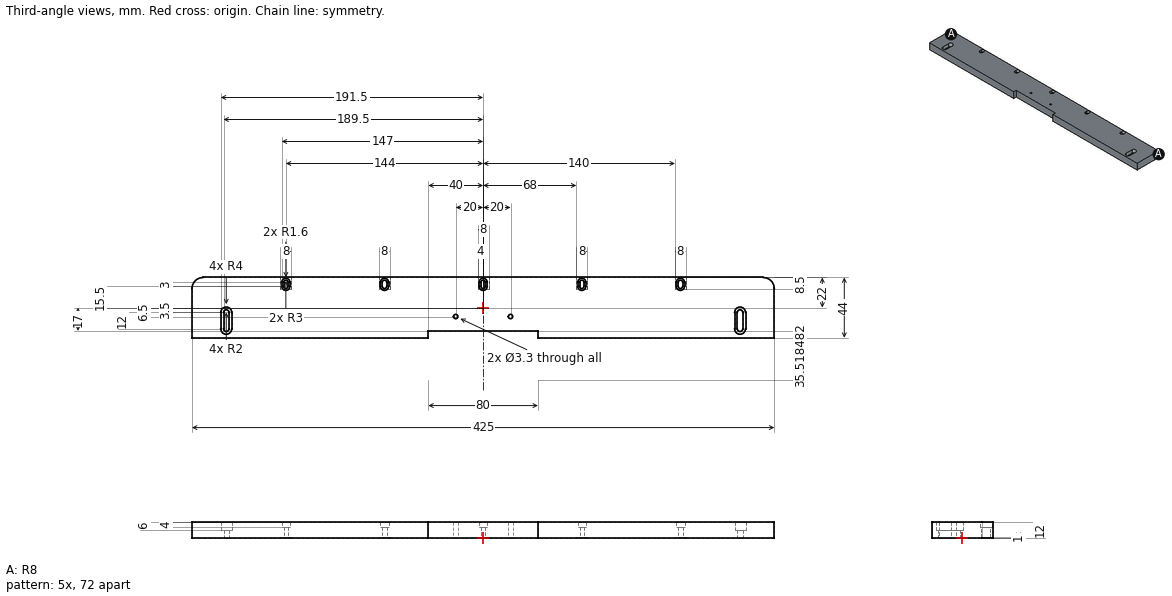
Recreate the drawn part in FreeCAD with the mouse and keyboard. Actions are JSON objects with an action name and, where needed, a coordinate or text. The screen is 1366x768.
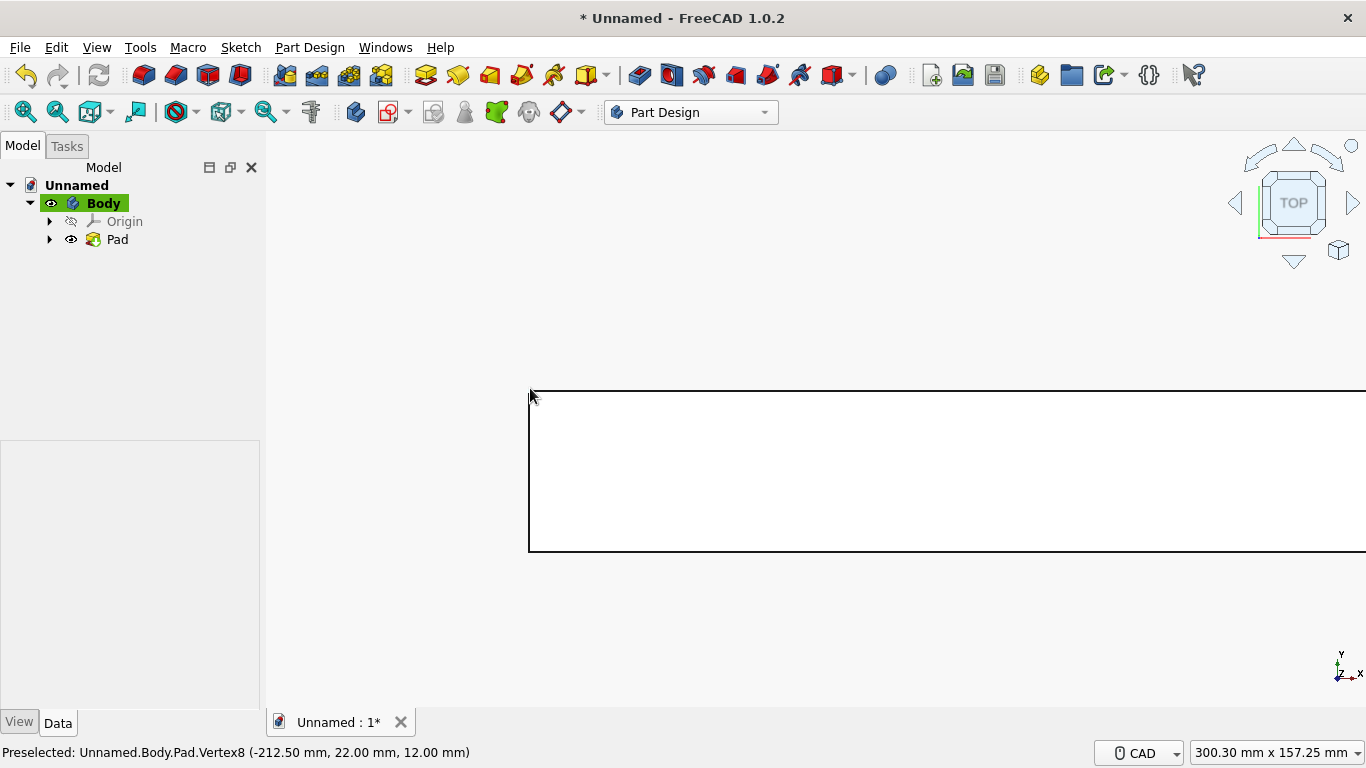
{"action": "key", "text": "v f"}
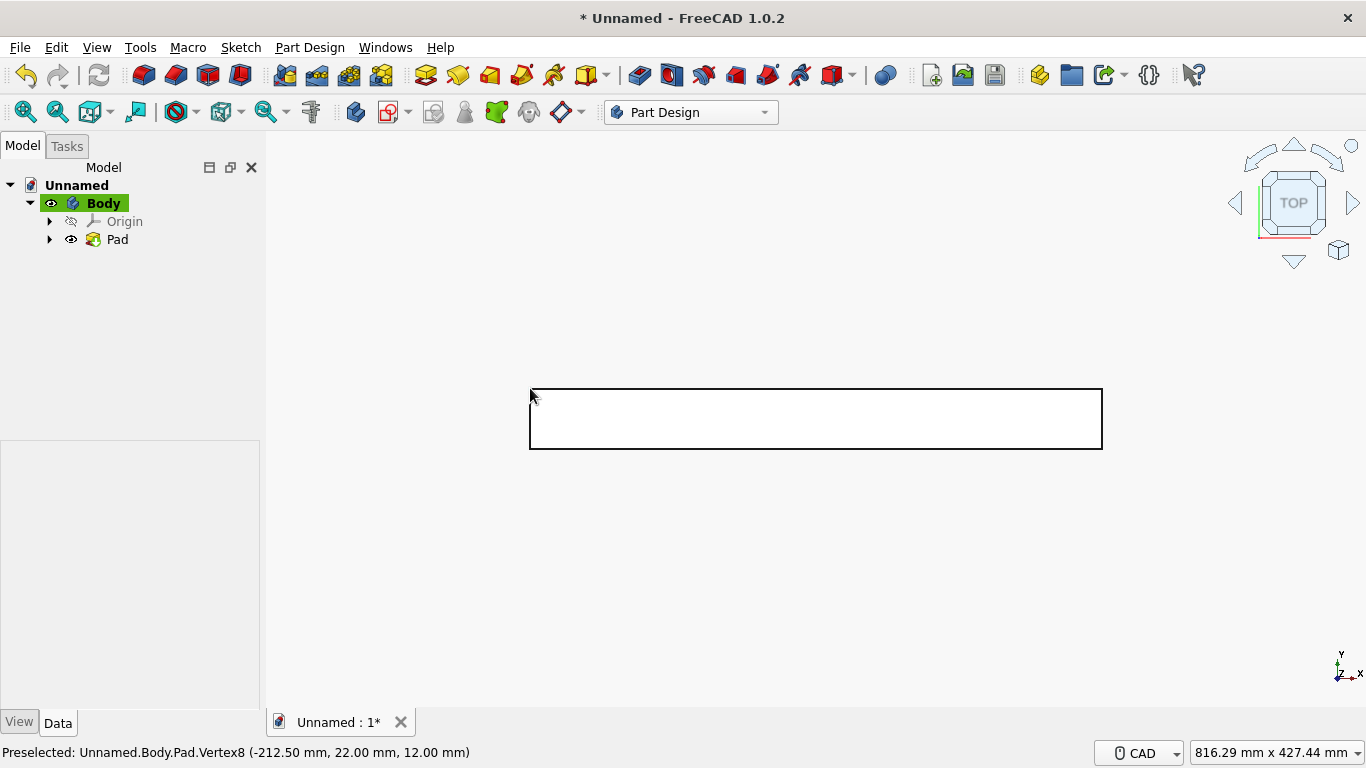
{"action": "key", "text": "1"}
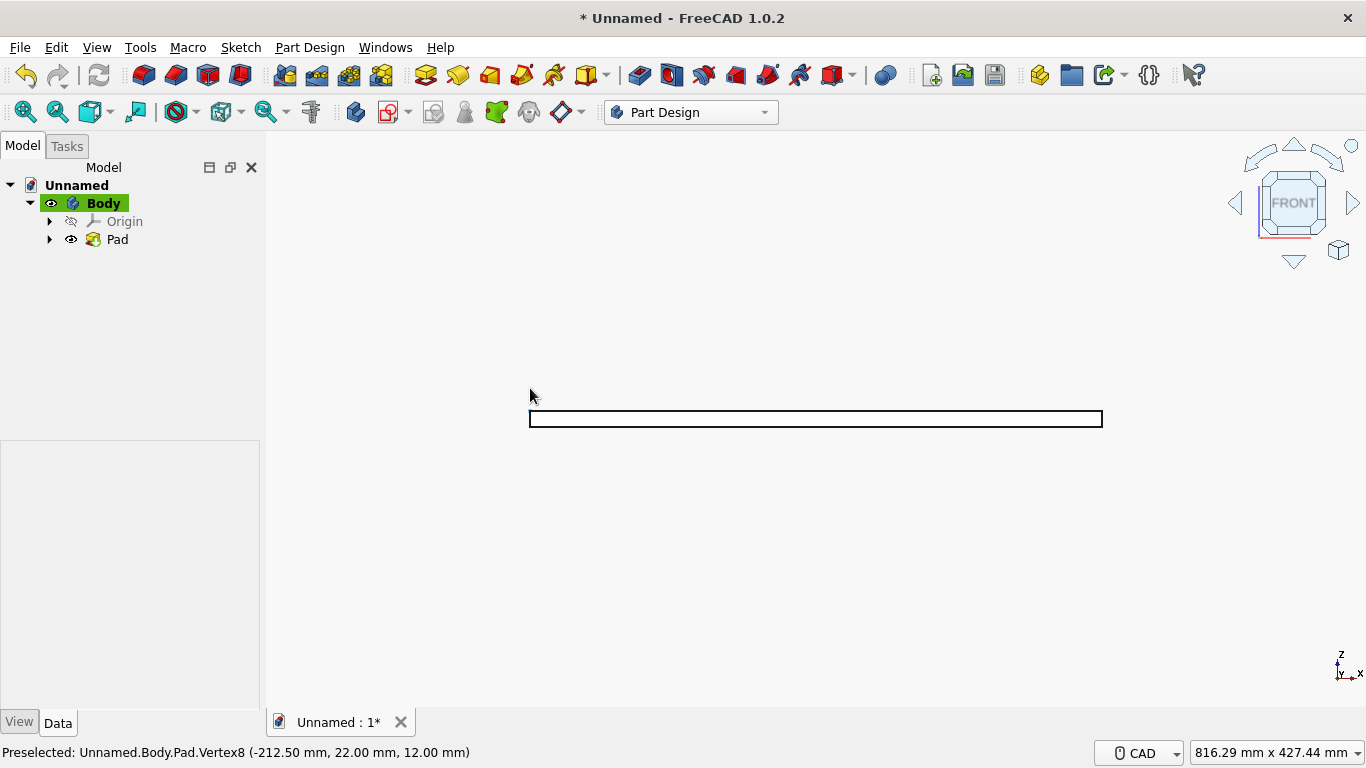
{"action": "scroll", "coordinate": [530, 418], "scroll_direction": "up", "scroll_amount": 5}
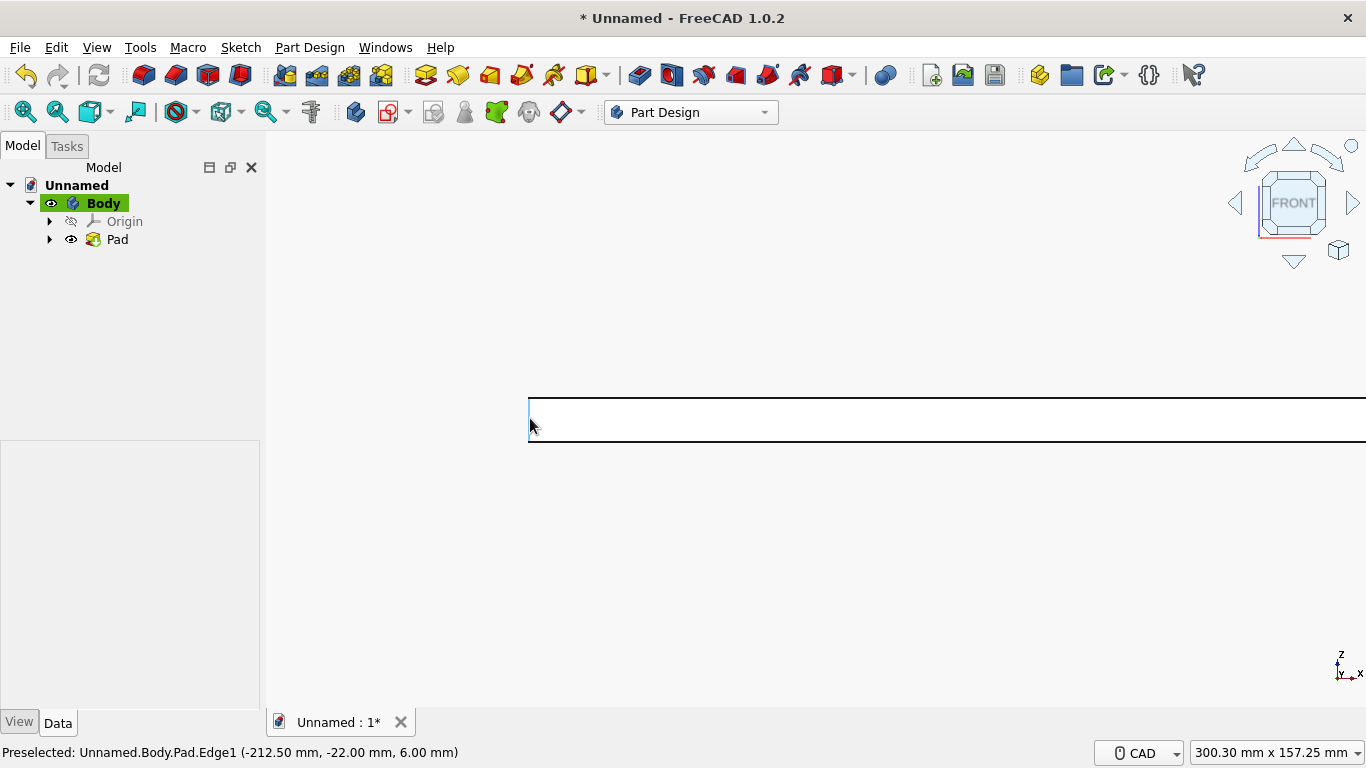
{"action": "left_click", "coordinate": [26, 112]}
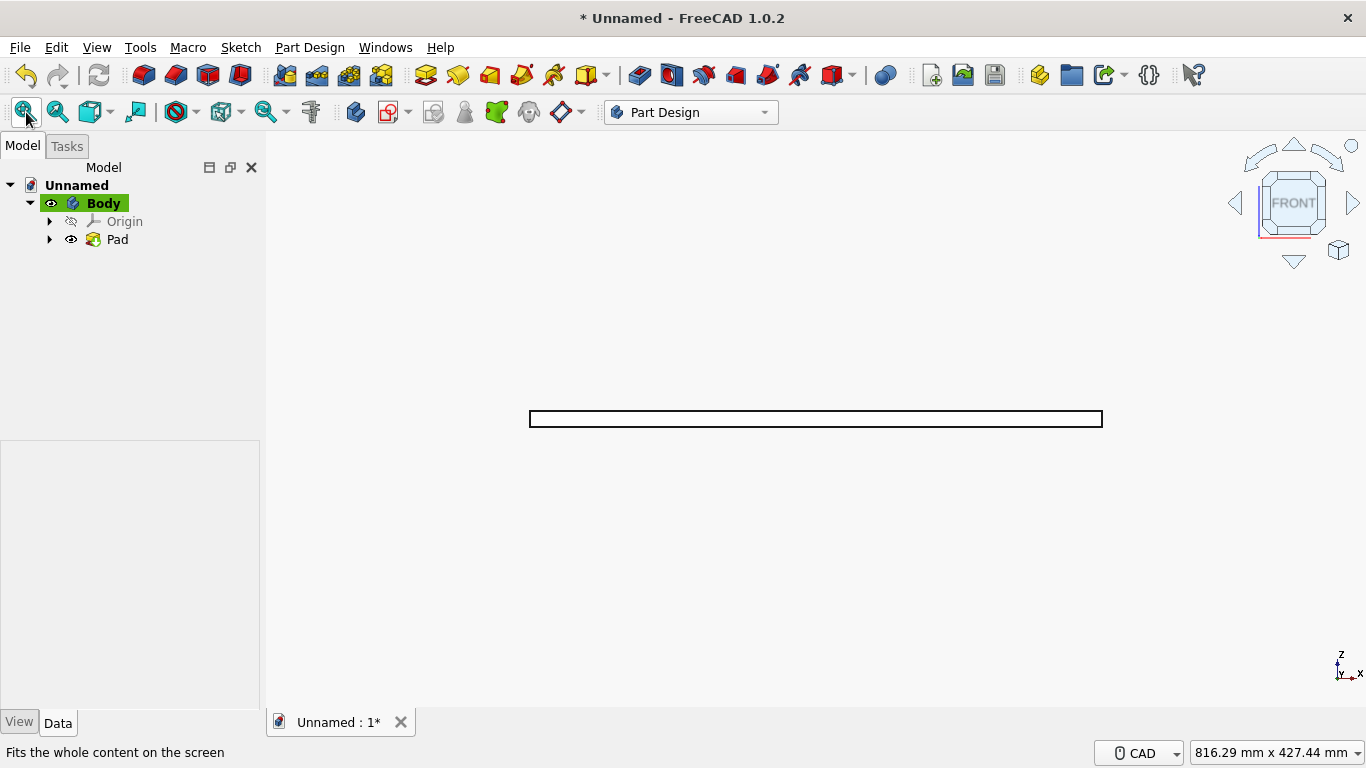
{"action": "key", "text": "3"}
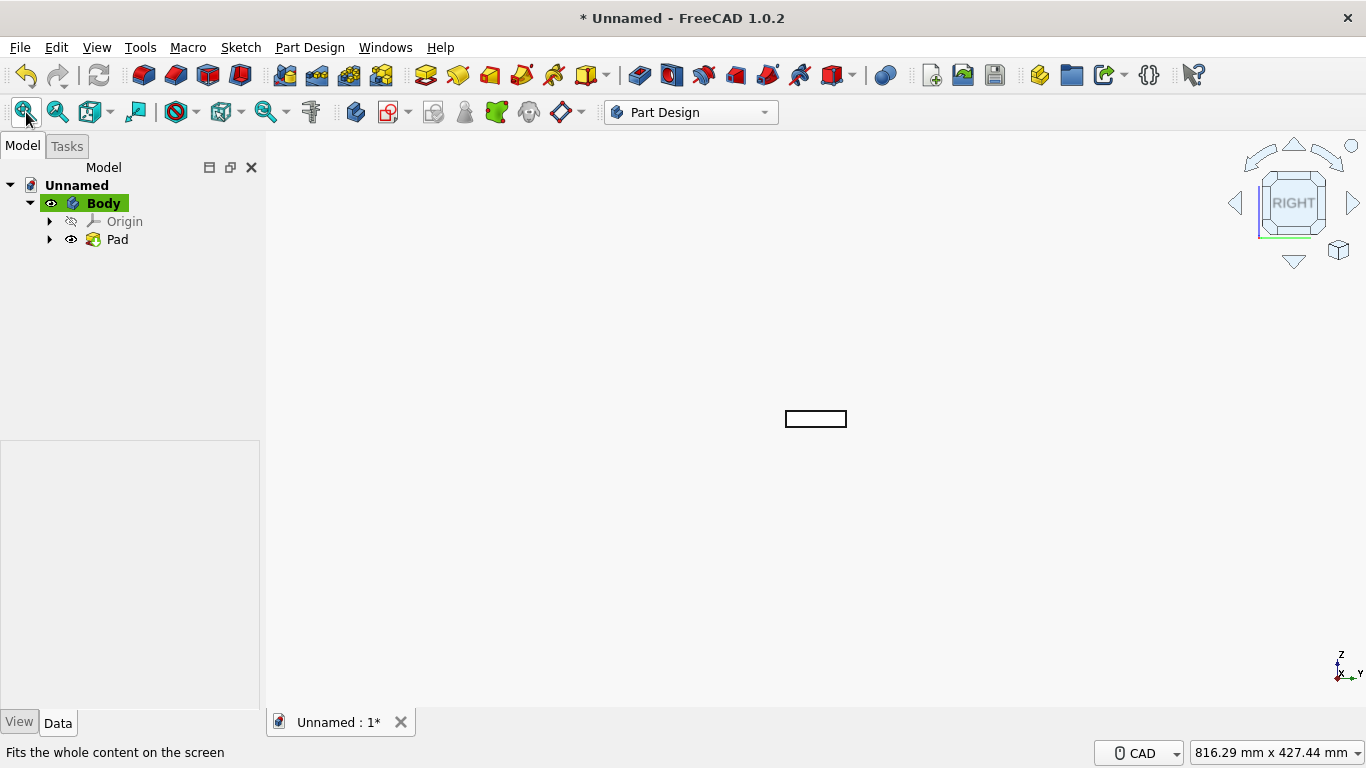
{"action": "left_click", "coordinate": [26, 112]}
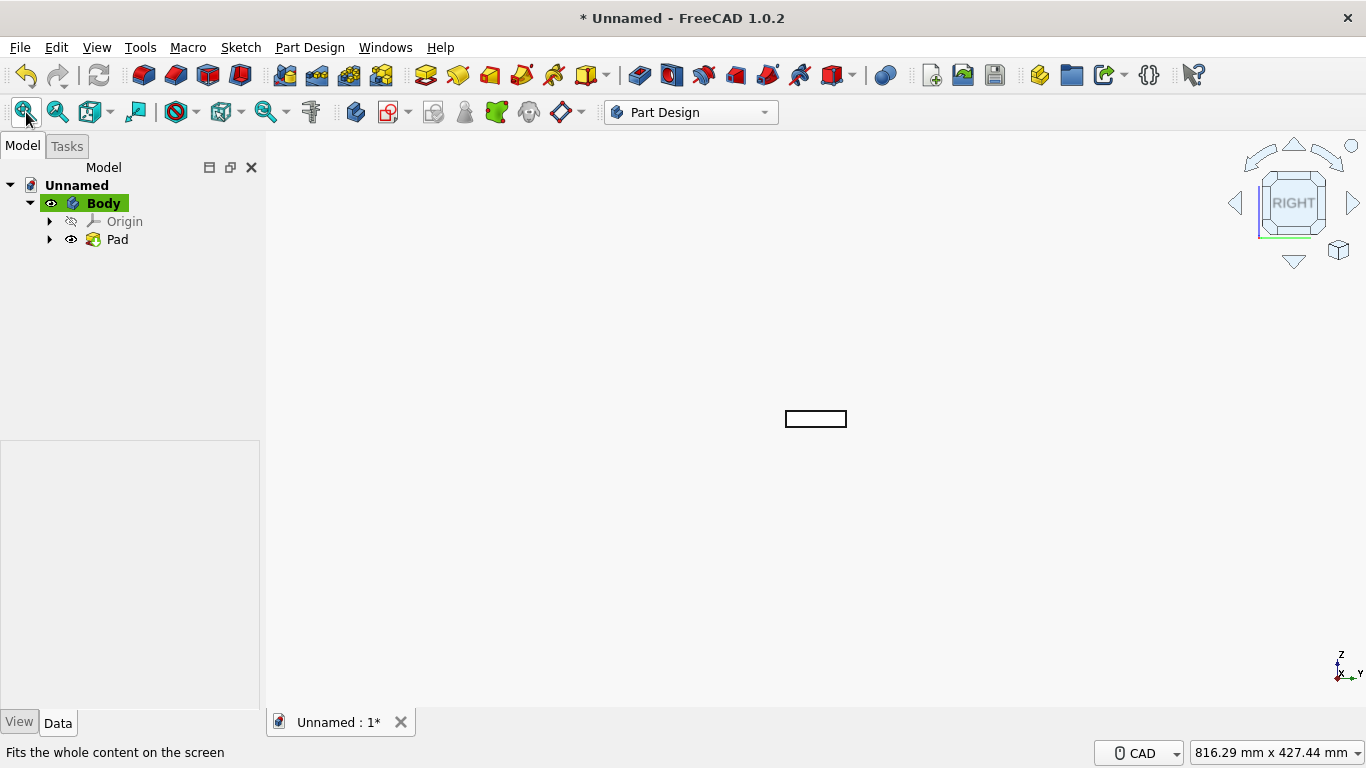
{"action": "left_click", "coordinate": [846, 418]}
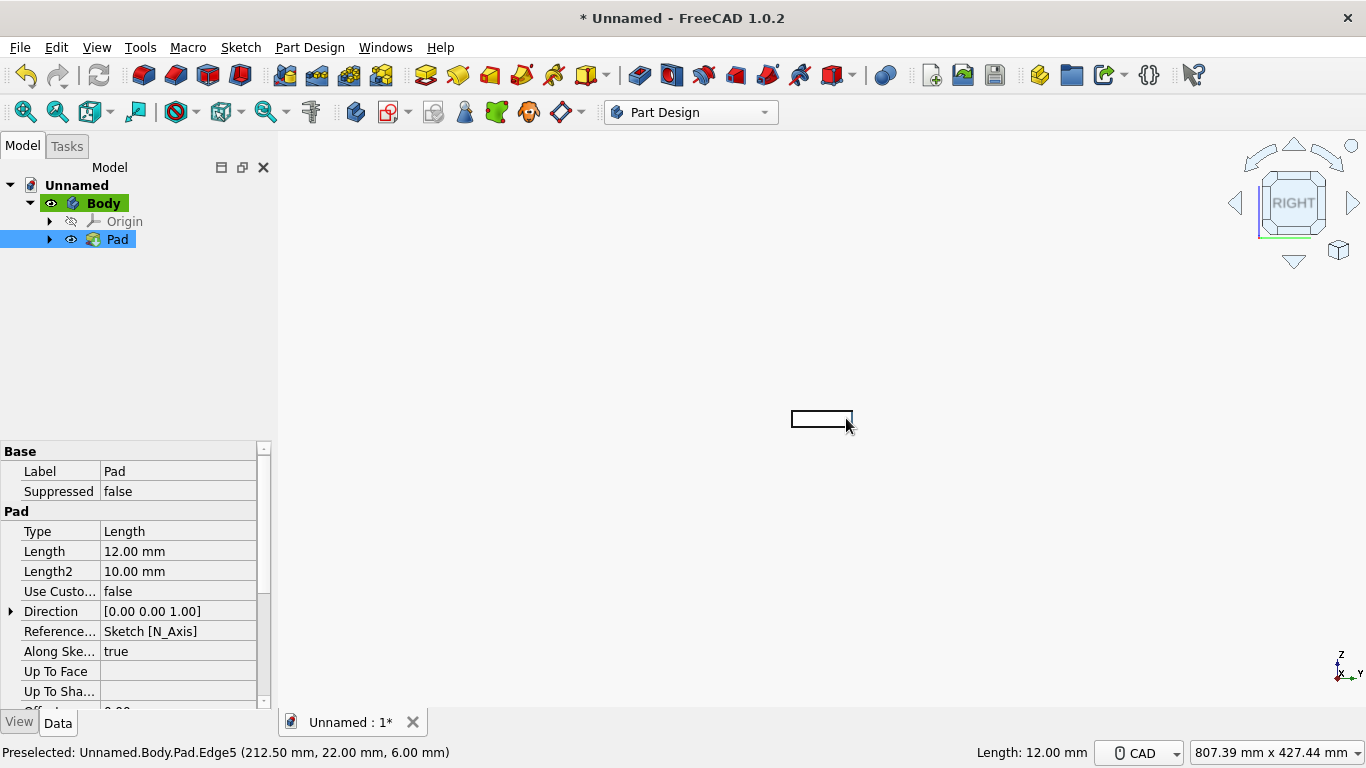
{"action": "scroll", "coordinate": [852, 418], "scroll_direction": "up", "scroll_amount": 5}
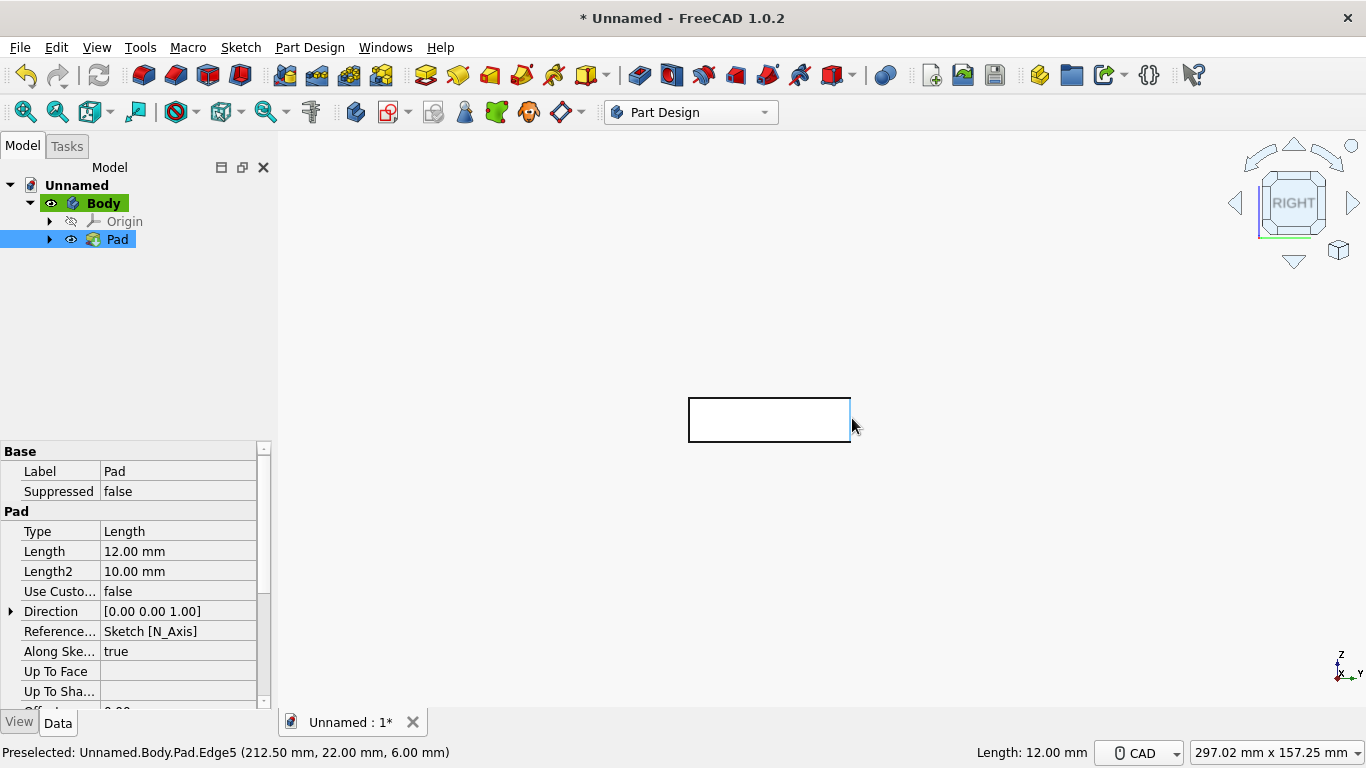
{"action": "left_click", "coordinate": [26, 112]}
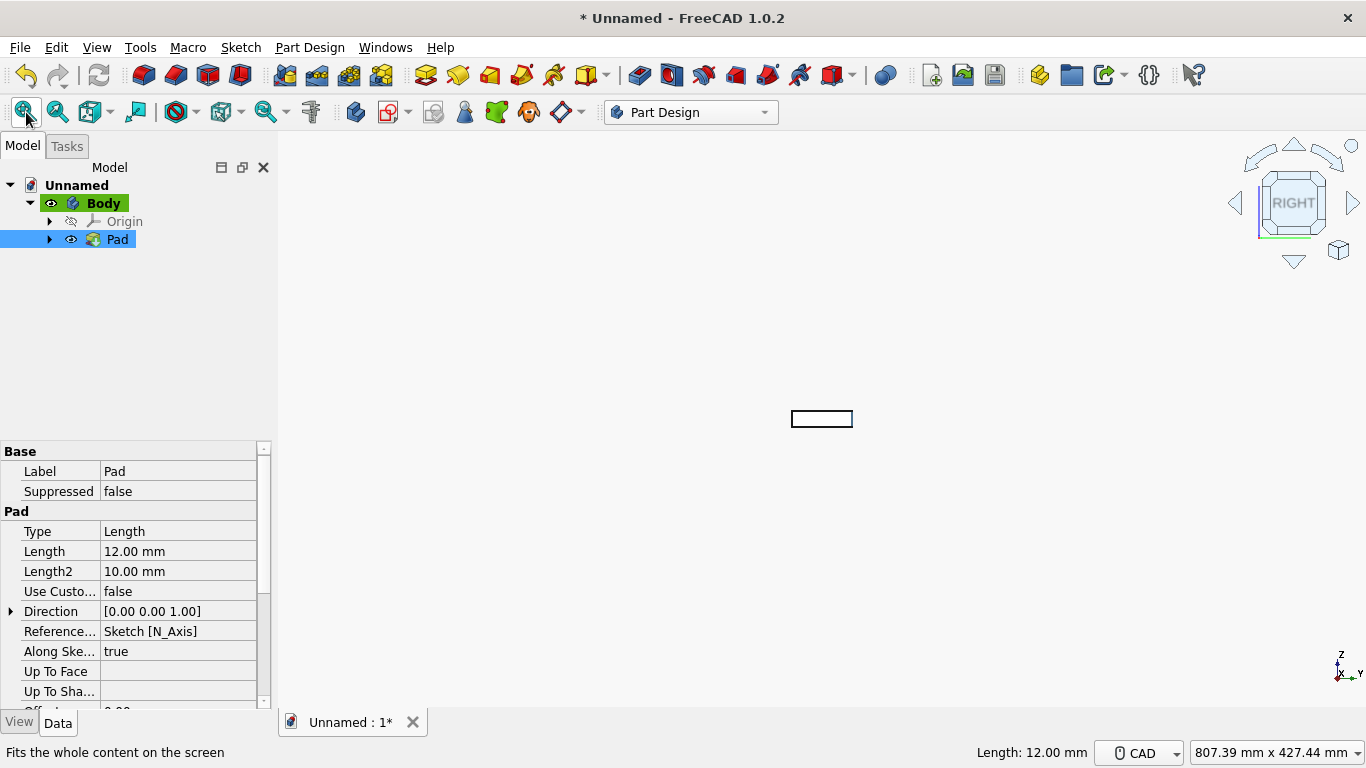
{"action": "key", "text": "5"}